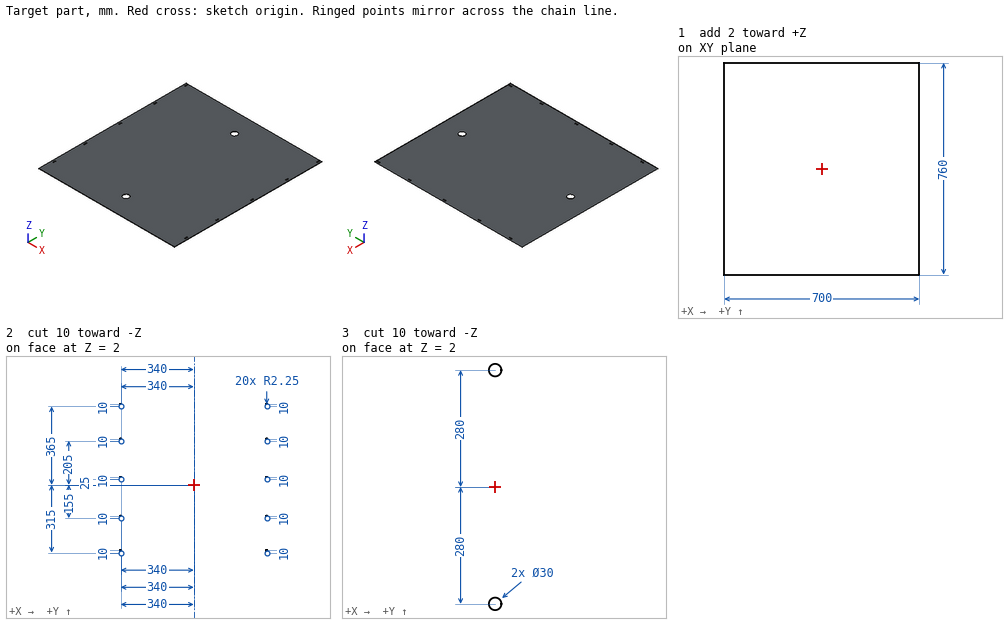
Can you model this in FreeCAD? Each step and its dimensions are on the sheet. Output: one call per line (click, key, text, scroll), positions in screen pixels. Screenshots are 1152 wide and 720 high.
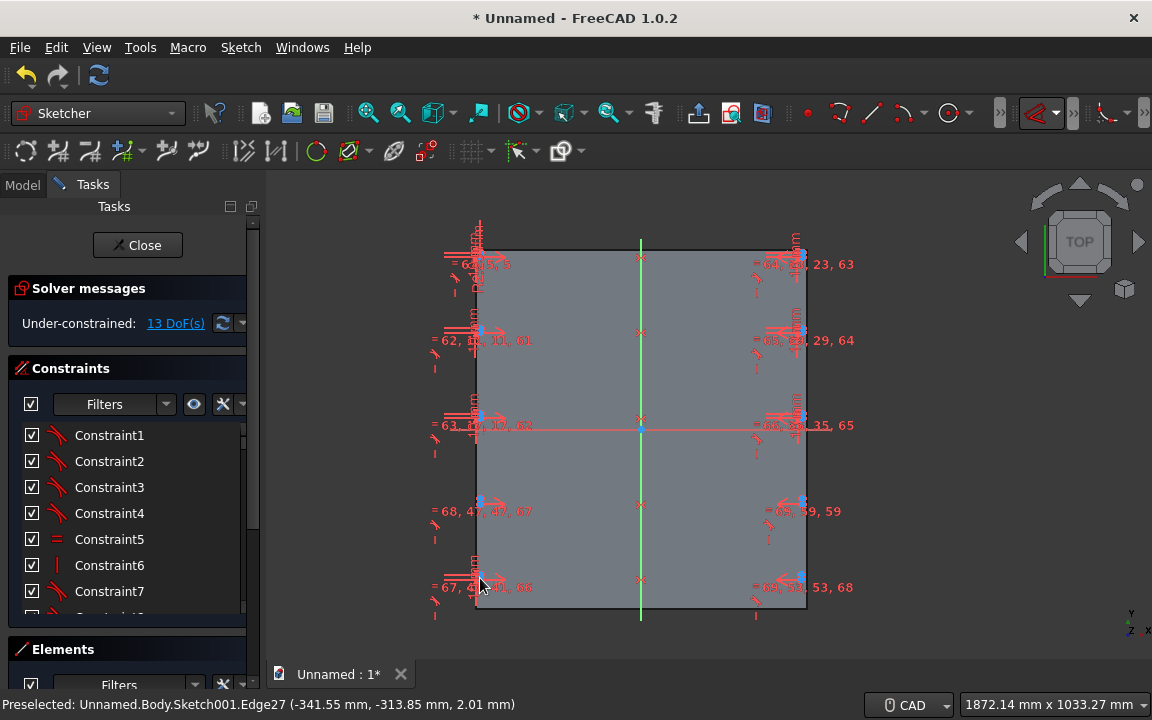
scroll(479, 503, up, 11)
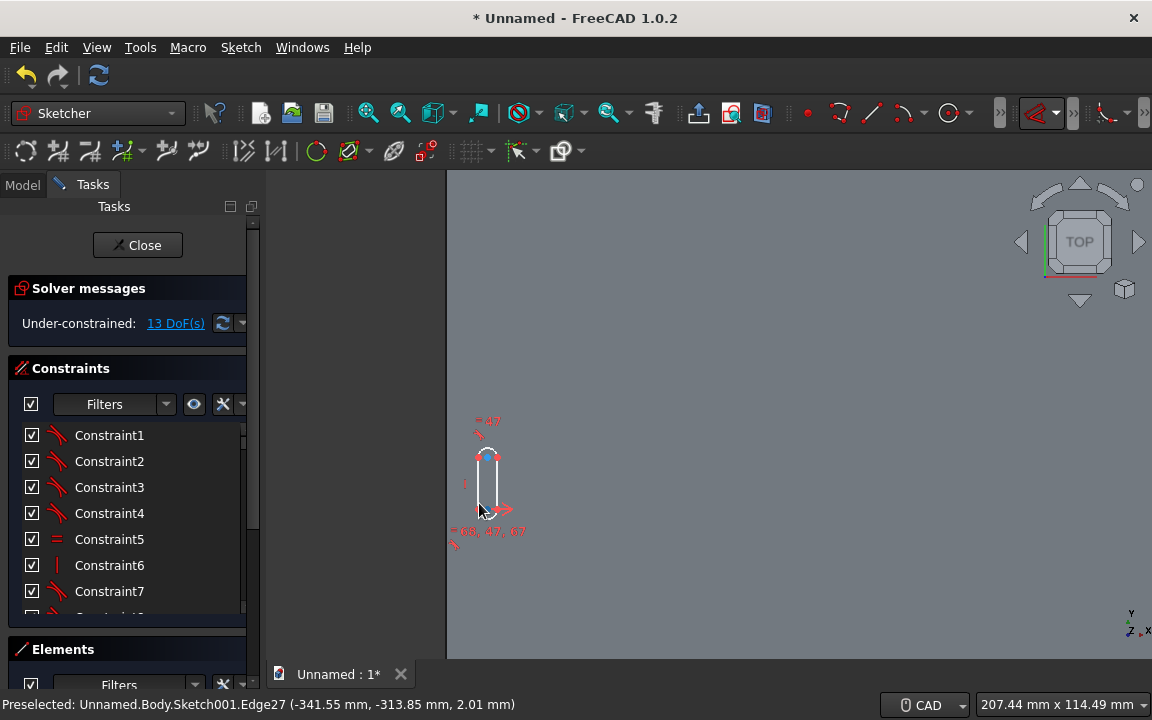
click(478, 494)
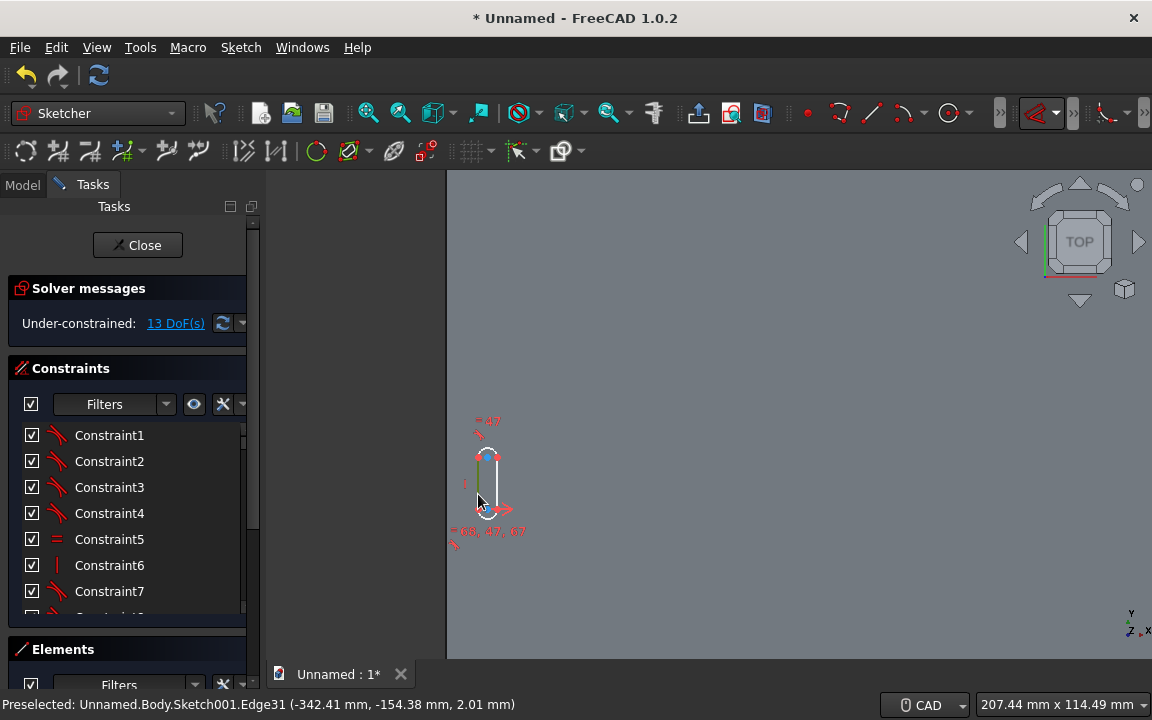
click(1058, 114)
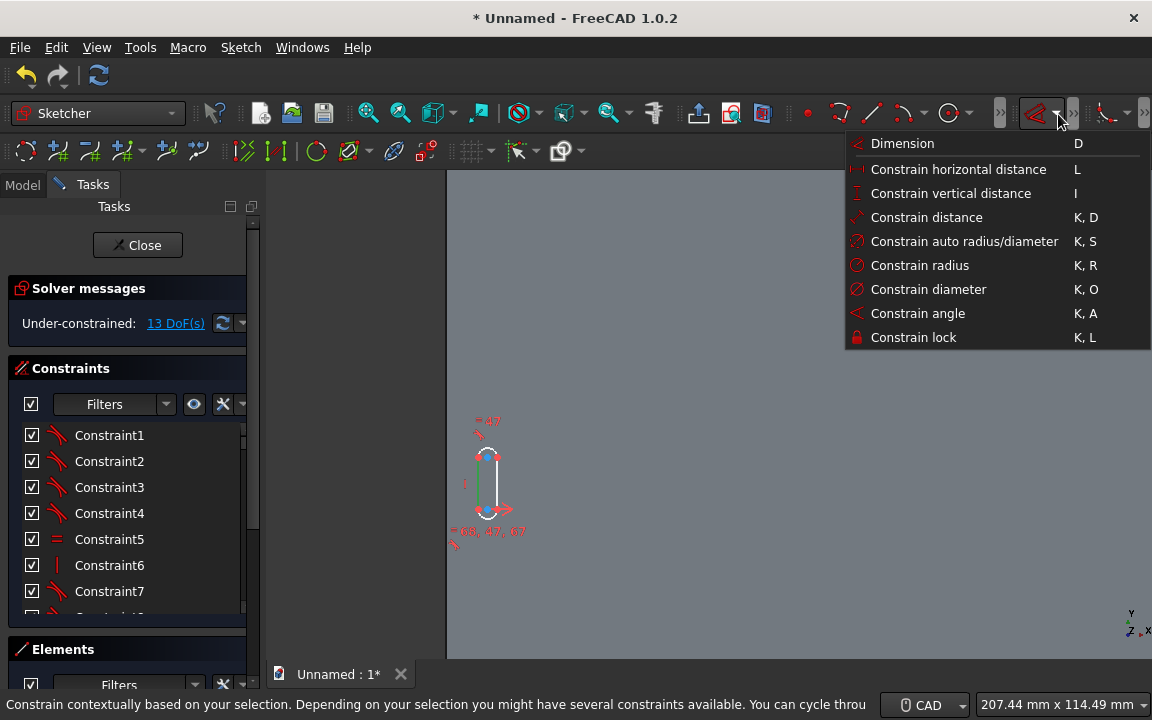
click(998, 193)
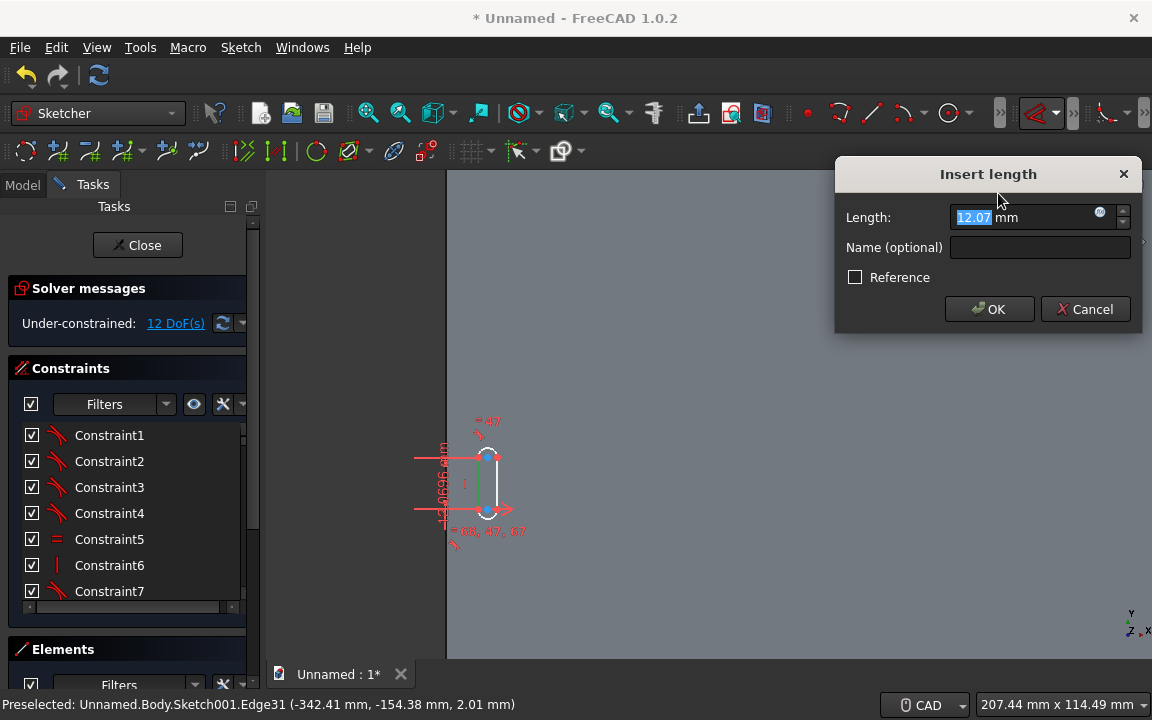
text(10)
key(Return)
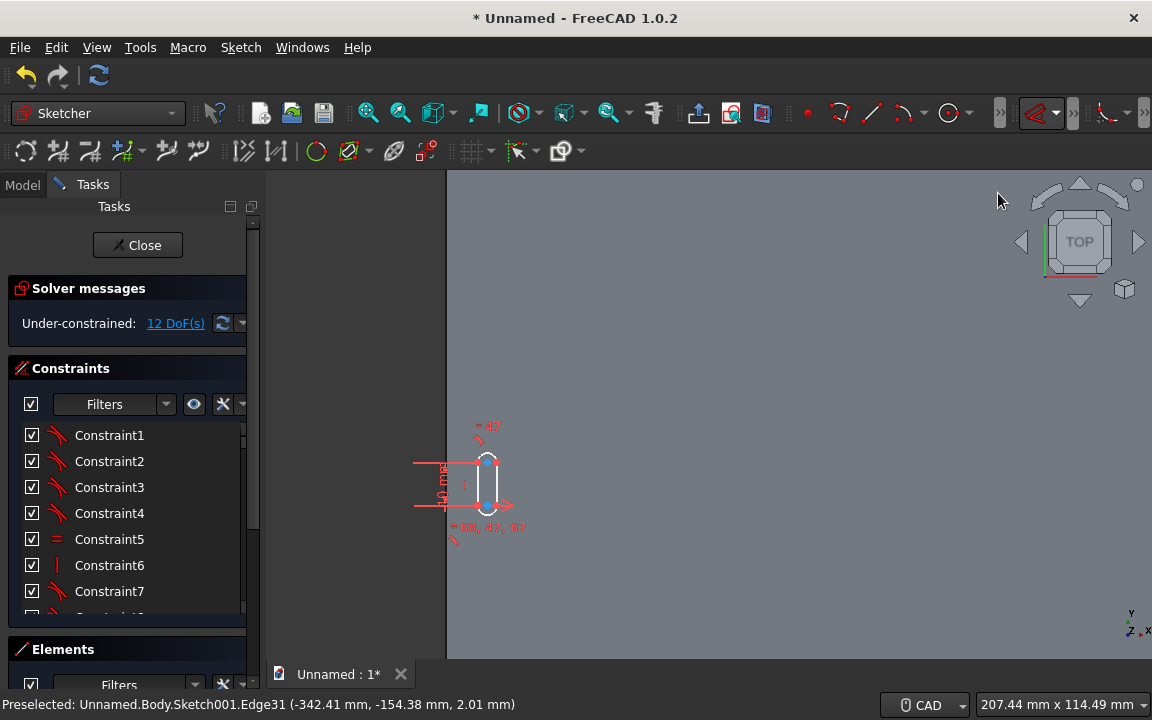
scroll(479, 503, down, 11)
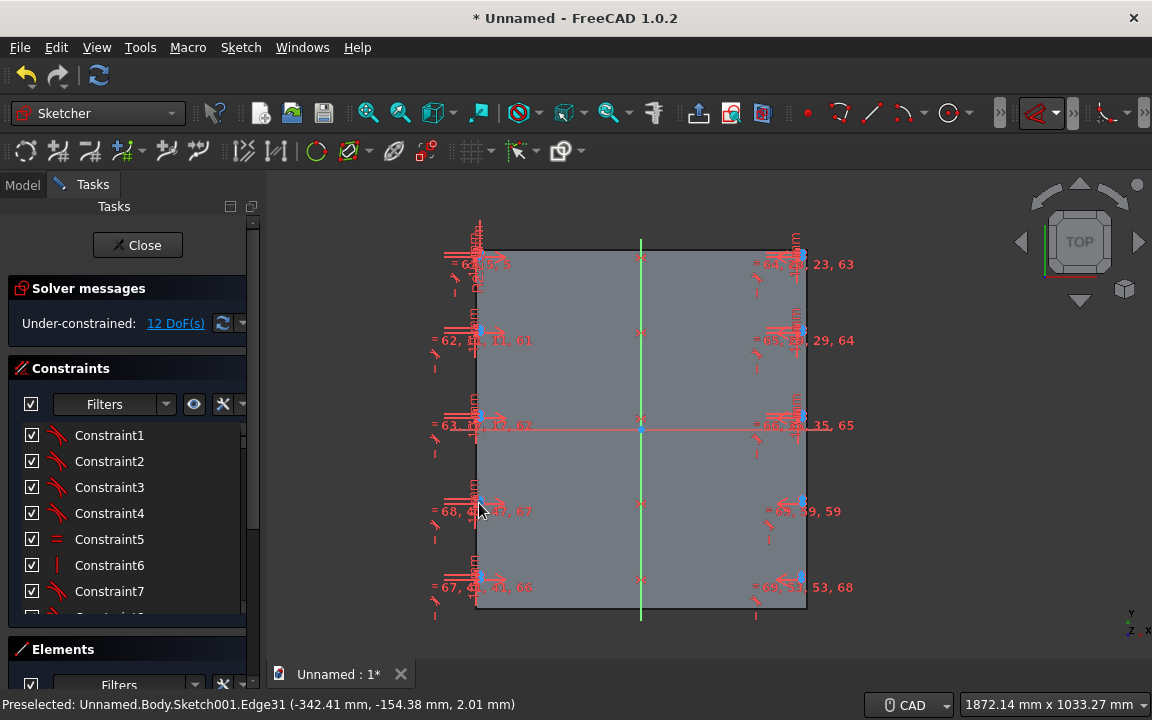
scroll(801, 578, up, 11)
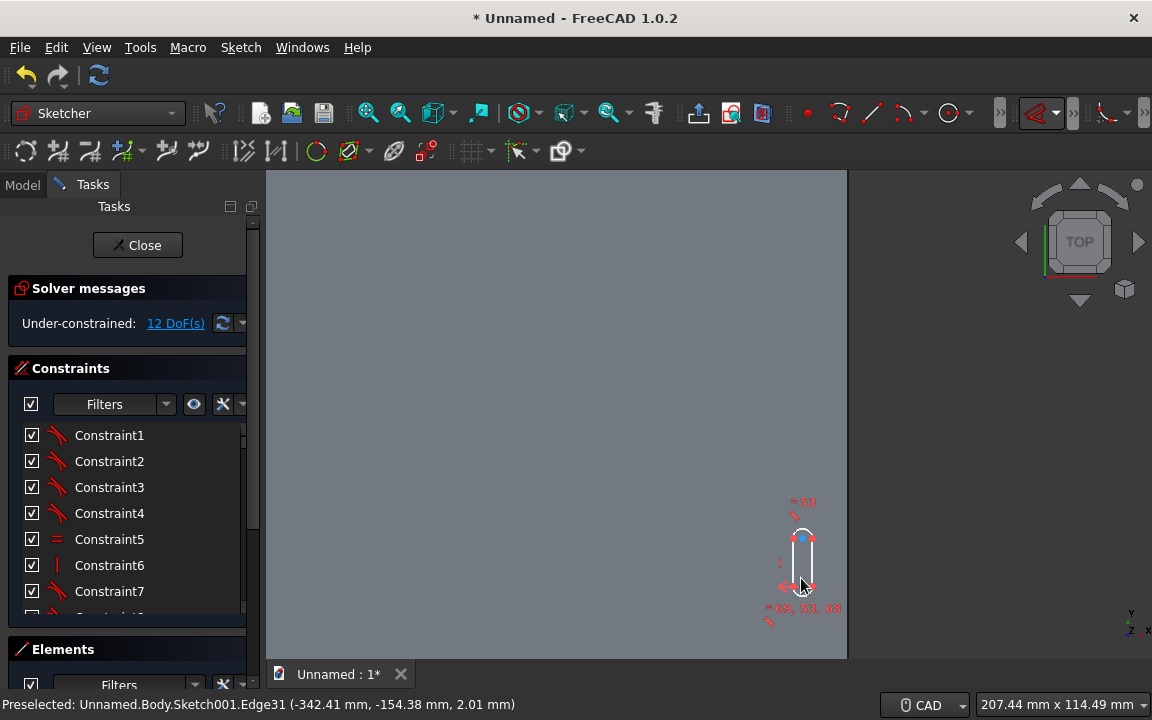
click(793, 572)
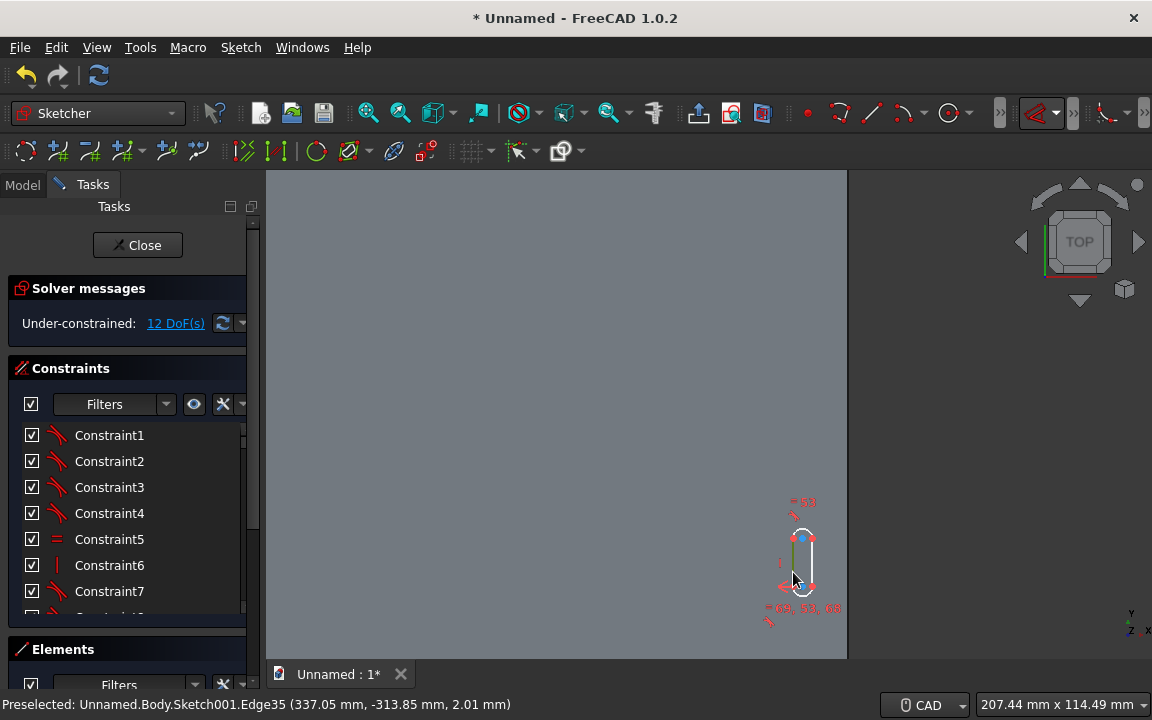
key(i)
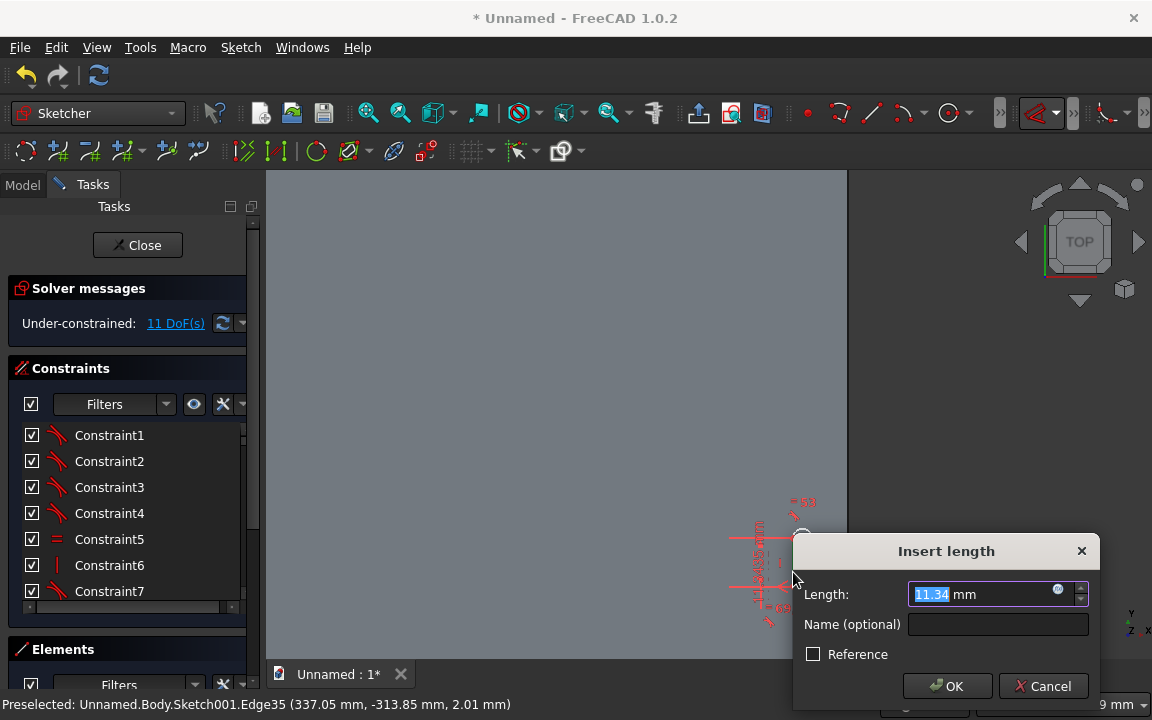
text(10)
key(Return)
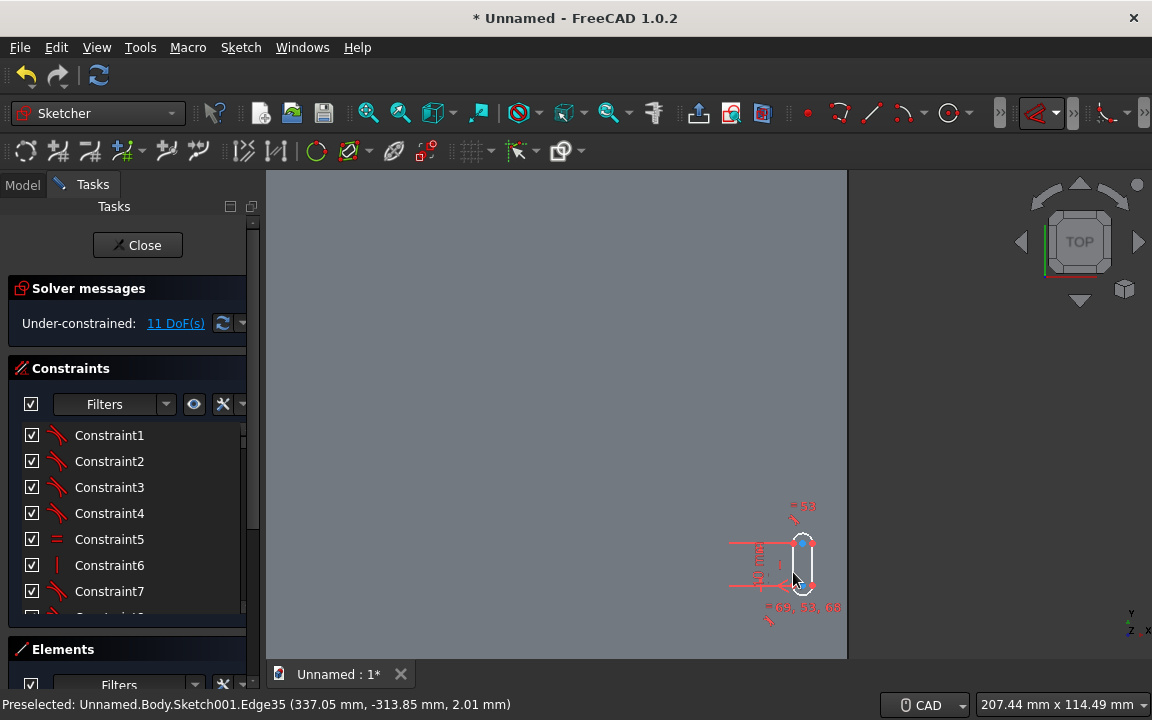
scroll(801, 578, down, 11)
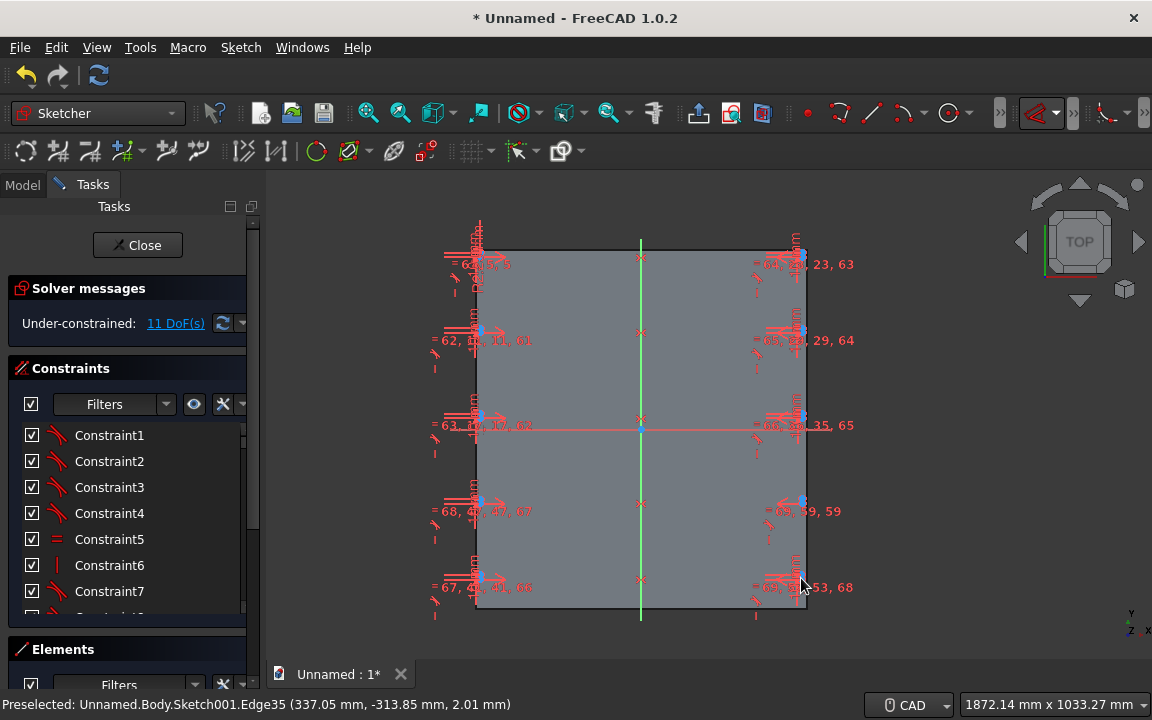
scroll(801, 502, up, 11)